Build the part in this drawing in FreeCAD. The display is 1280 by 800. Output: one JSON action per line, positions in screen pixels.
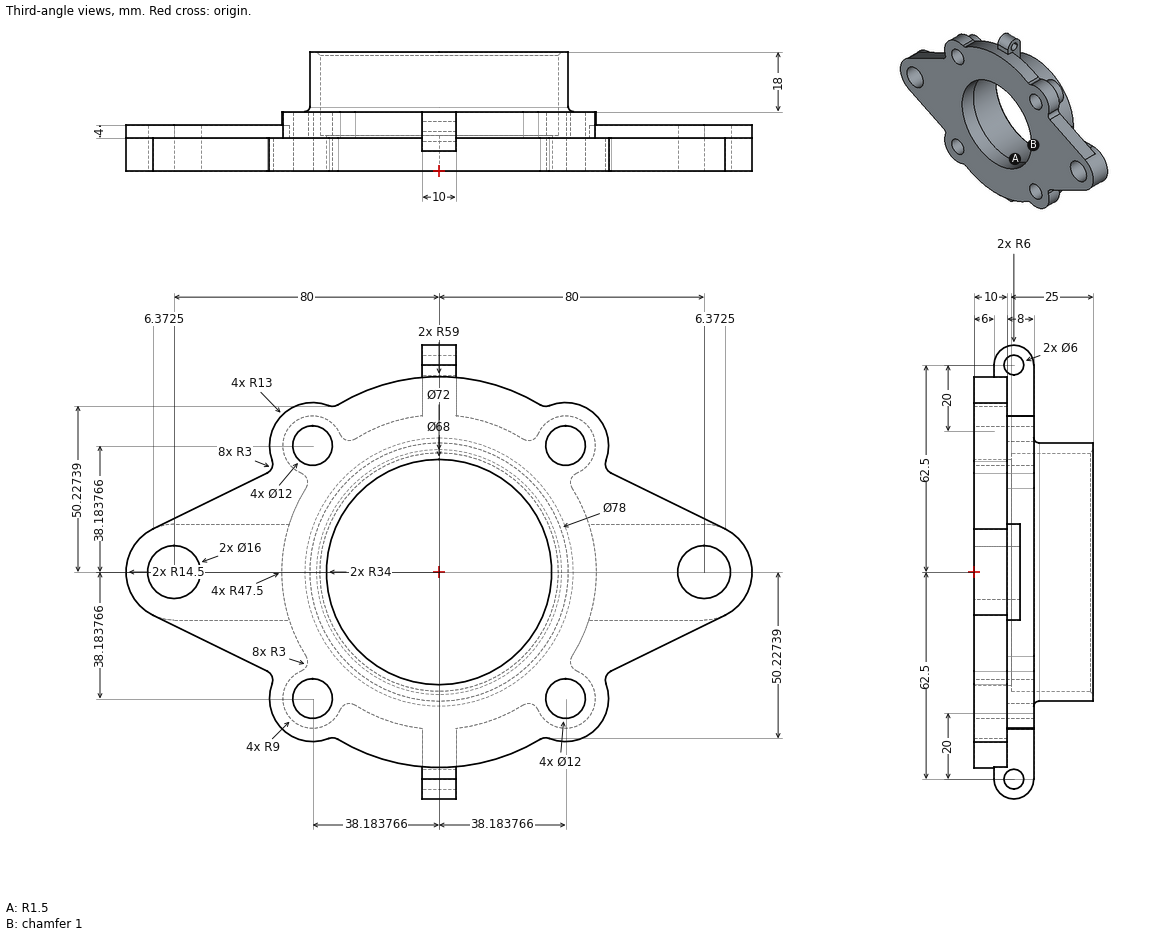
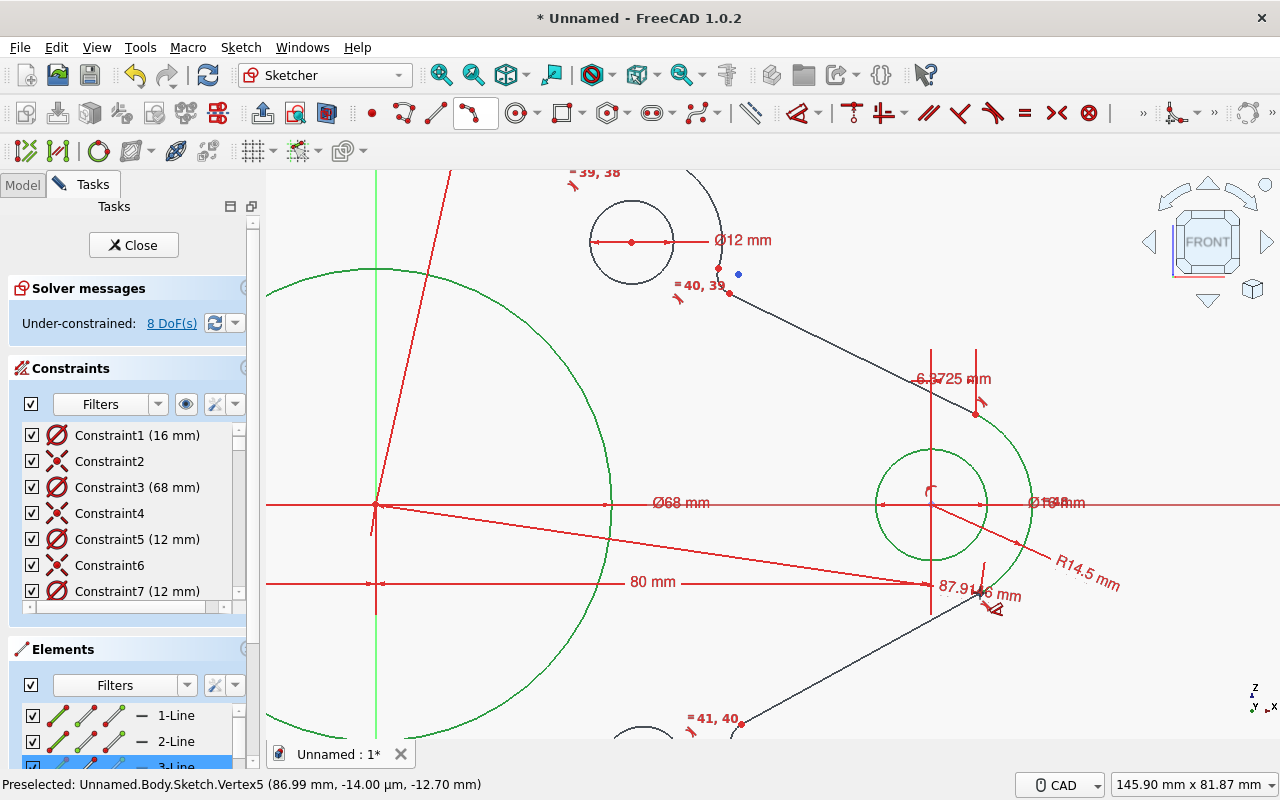
{"action": "left_click", "coordinate": [931, 505]}
{"action": "left_click", "coordinate": [956, 627]}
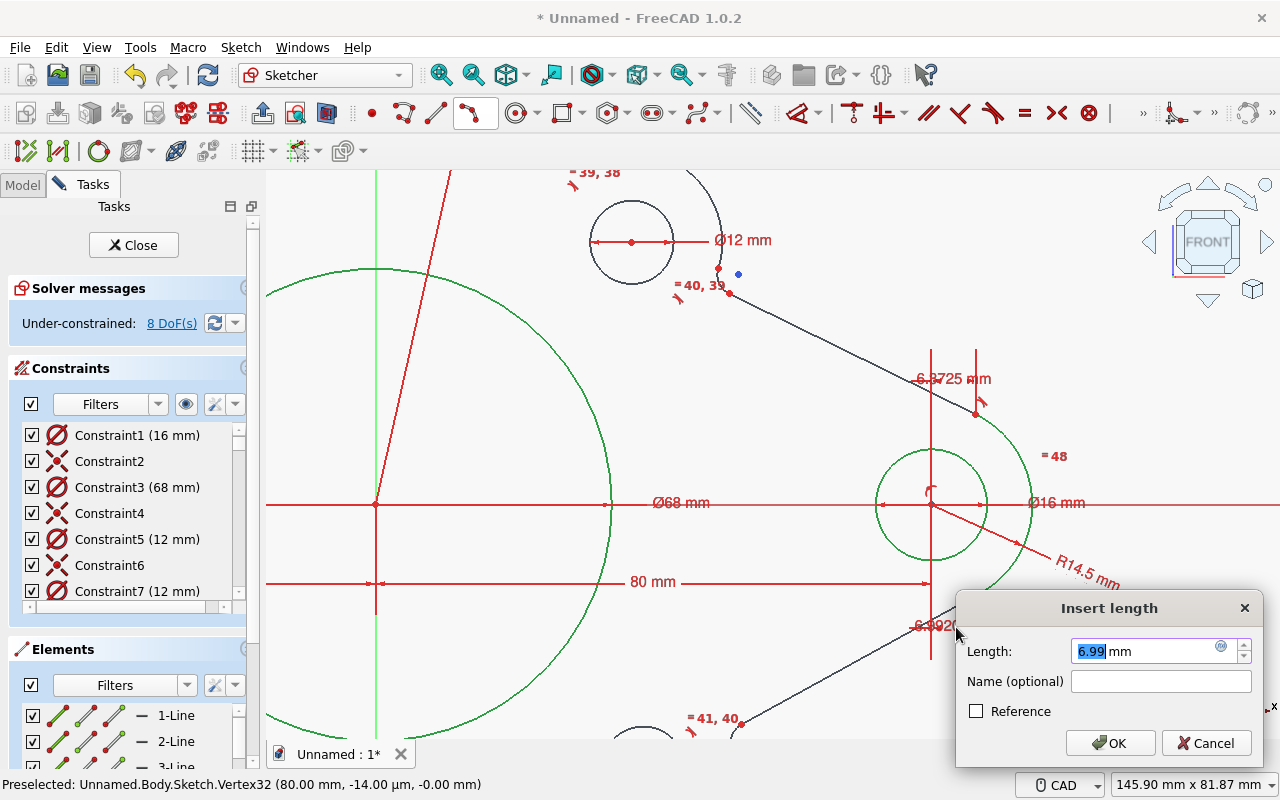
{"action": "type", "text": "6.3725"}
{"action": "key", "text": "Return"}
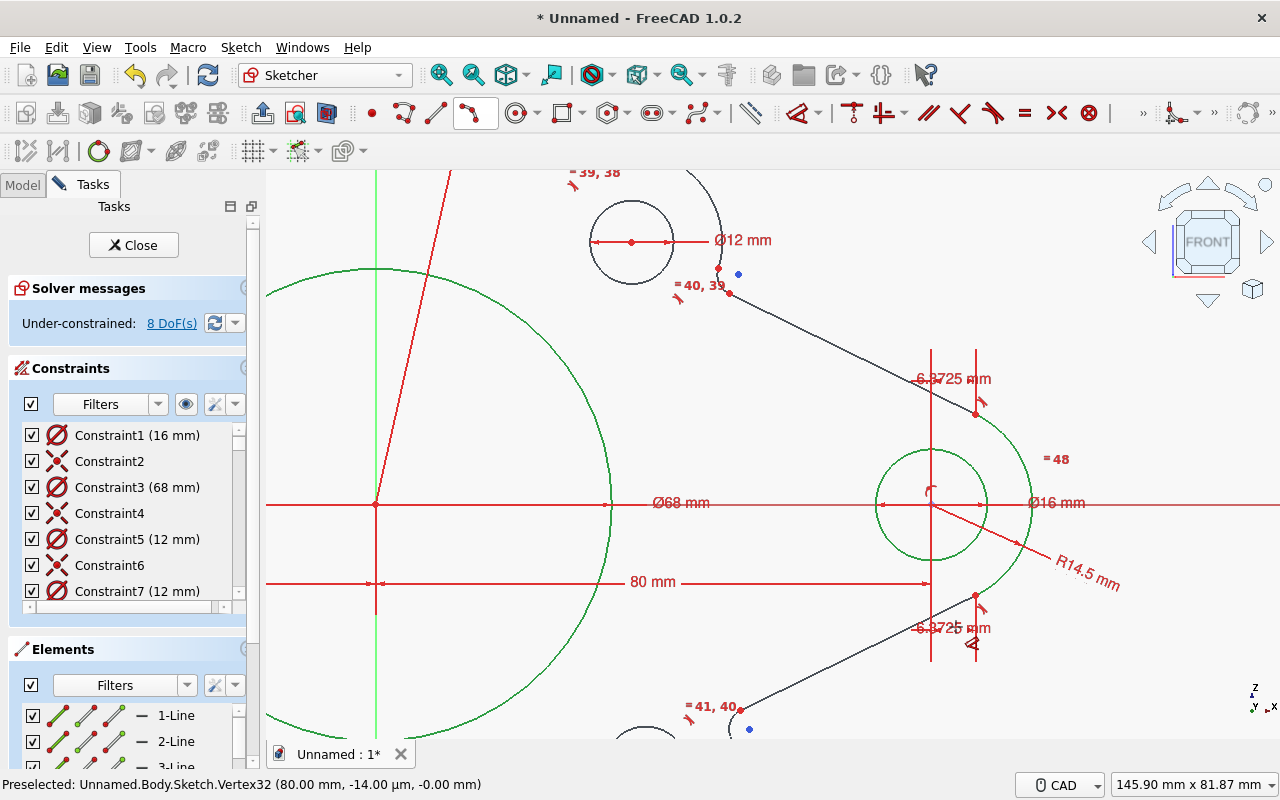
{"action": "scroll", "coordinate": [973, 413], "scroll_direction": "down", "scroll_amount": 4}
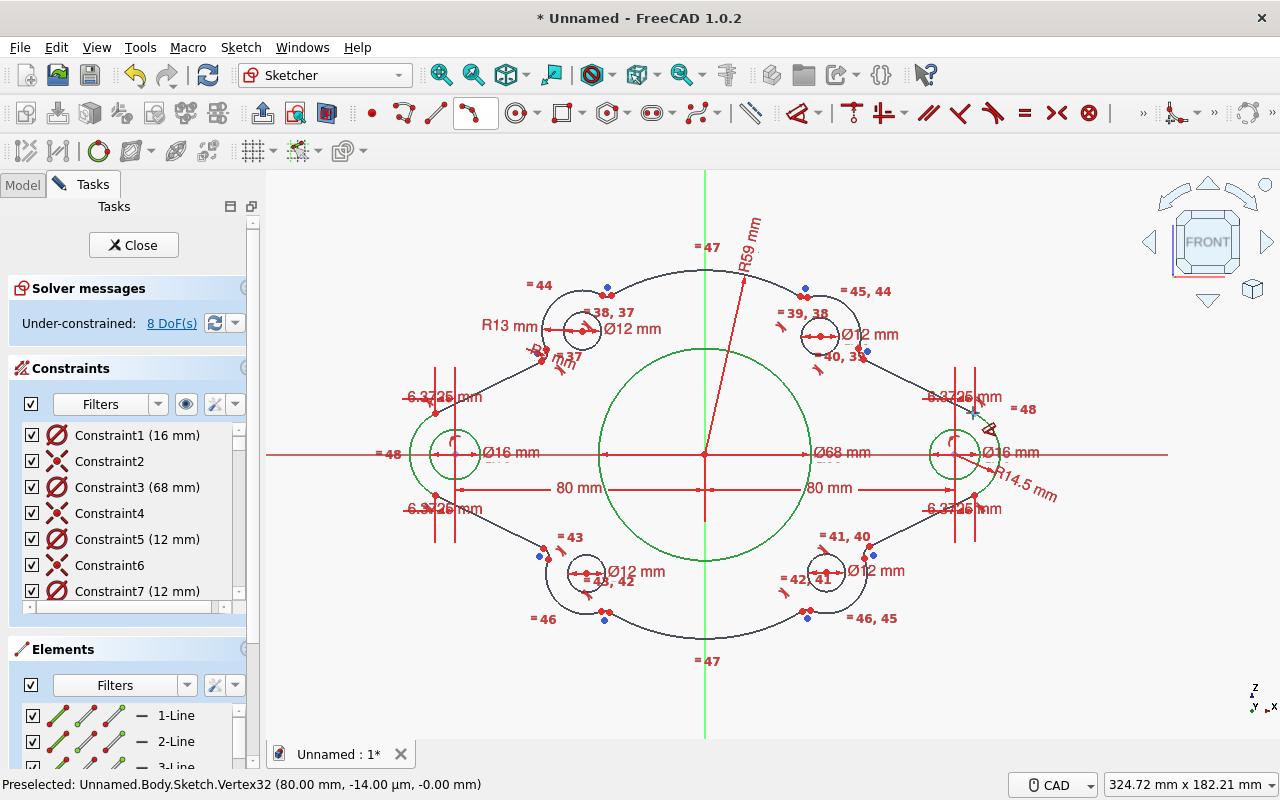
{"action": "scroll", "coordinate": [602, 296], "scroll_direction": "up", "scroll_amount": 2}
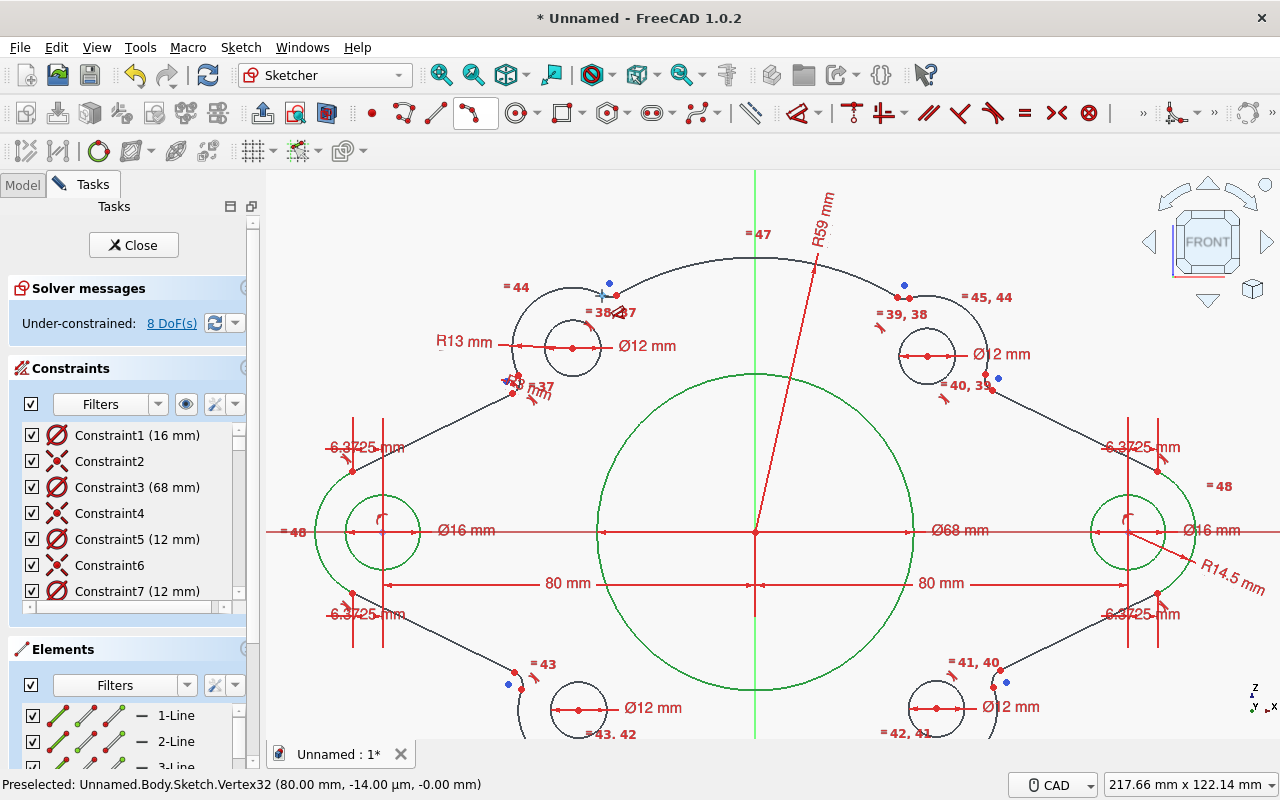
{"action": "left_click", "coordinate": [603, 295]}
{"action": "left_click", "coordinate": [569, 414]}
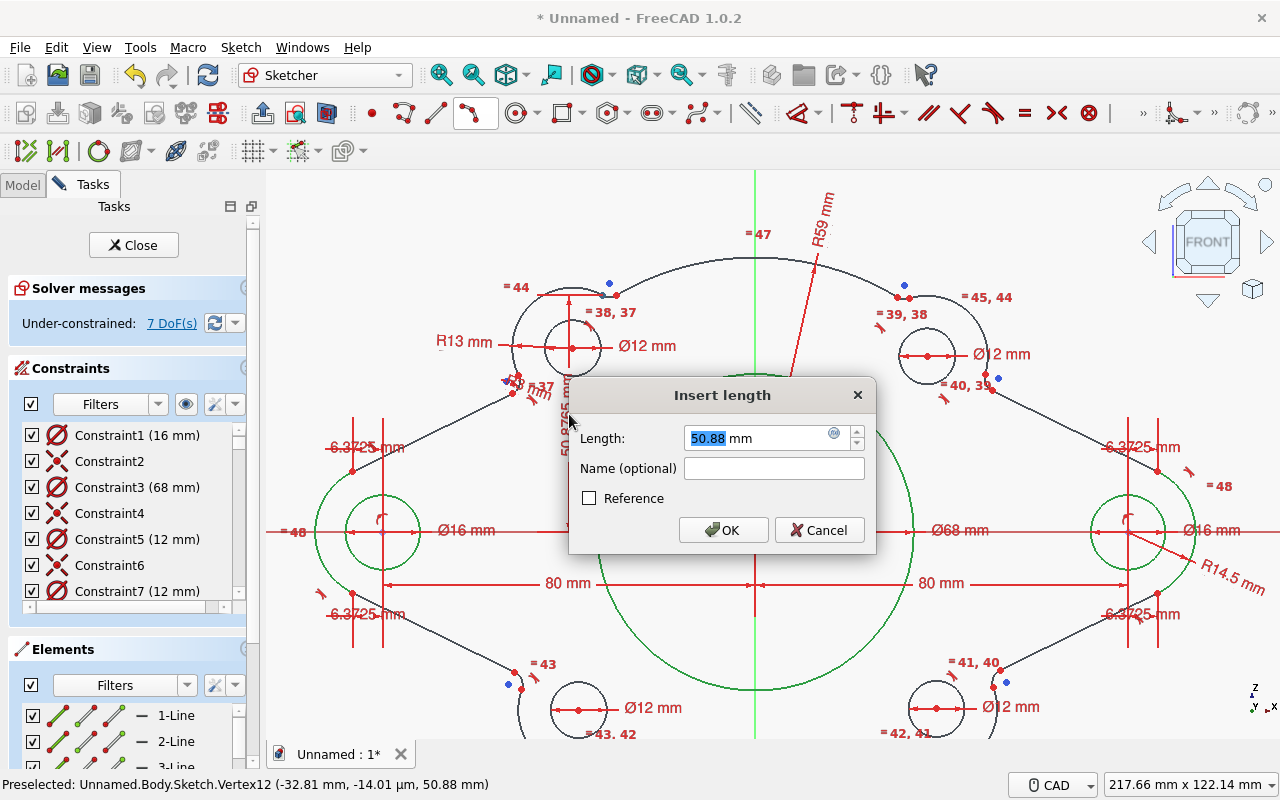
{"action": "type", "text": "50.22739"}
{"action": "key", "text": "Return"}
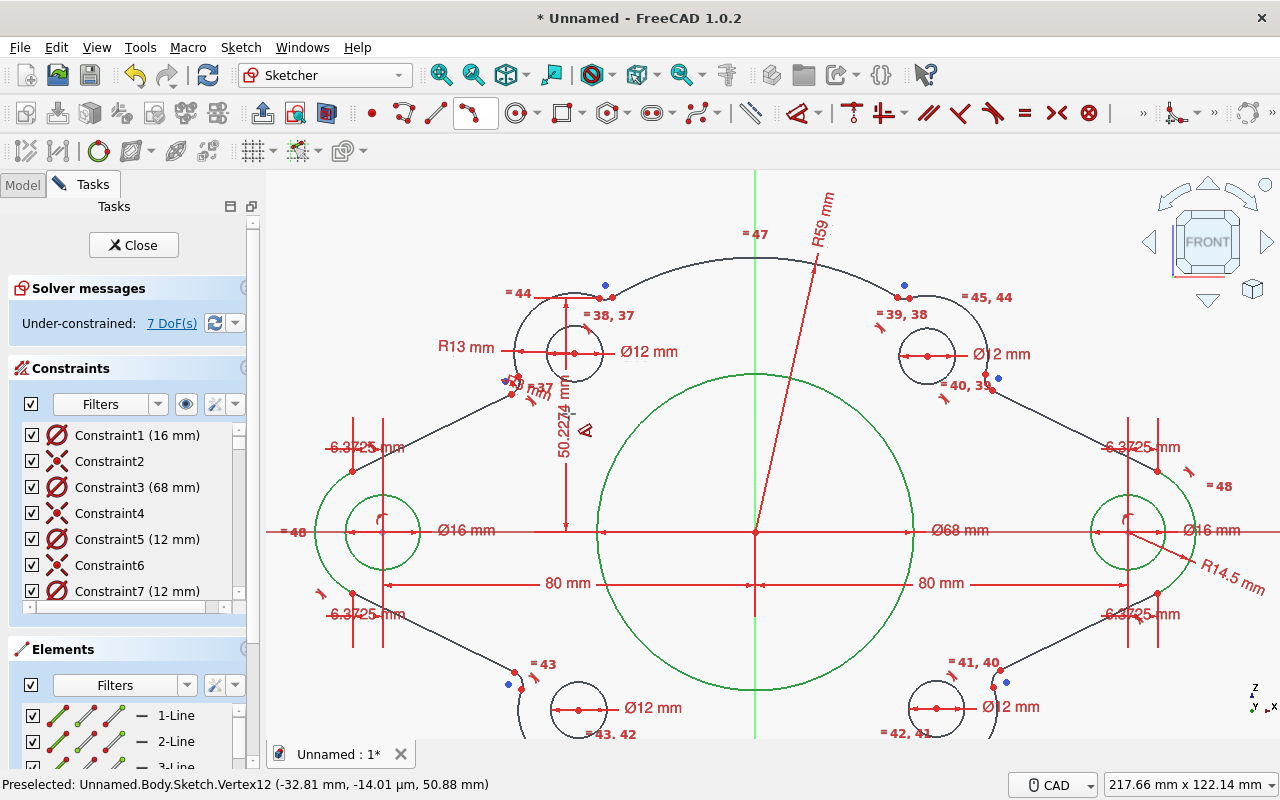
{"action": "left_click", "coordinate": [909, 299]}
{"action": "left_click", "coordinate": [943, 416]}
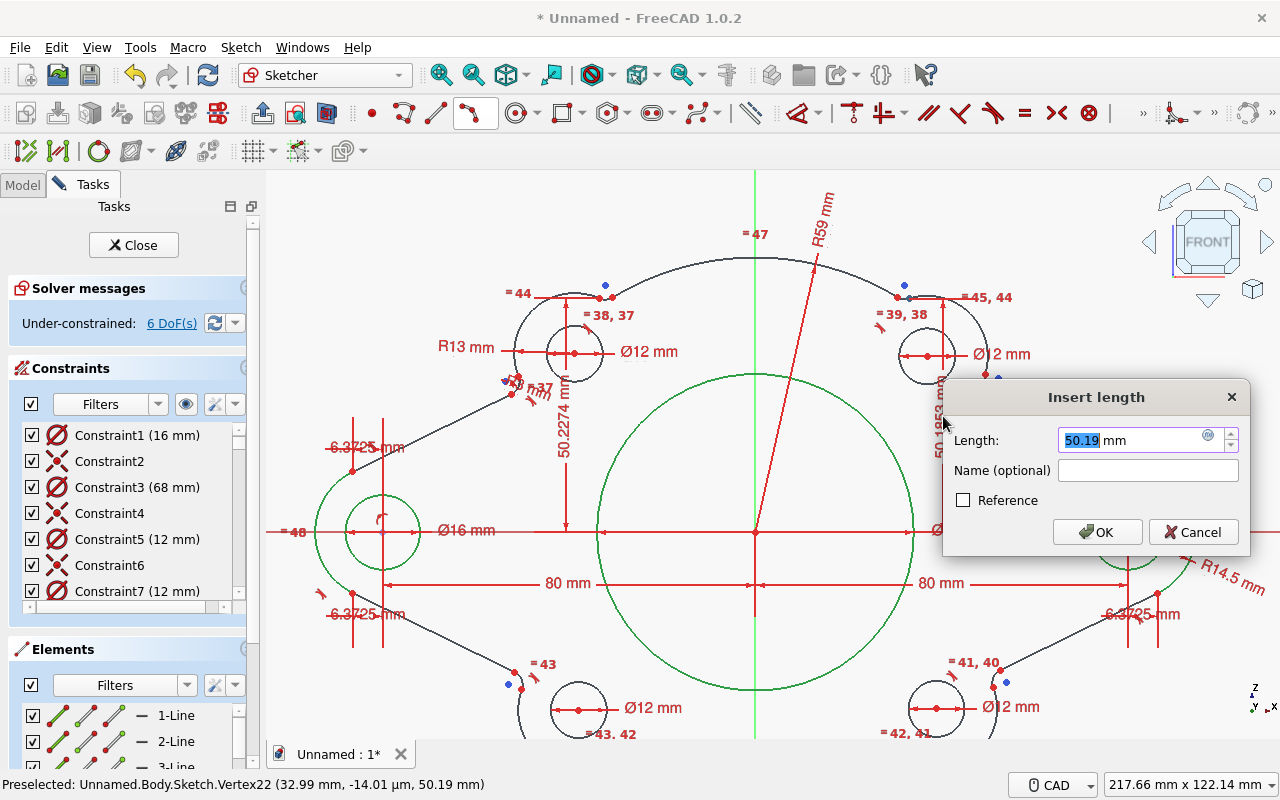
{"action": "type", "text": "50.22739"}
{"action": "key", "text": "Return"}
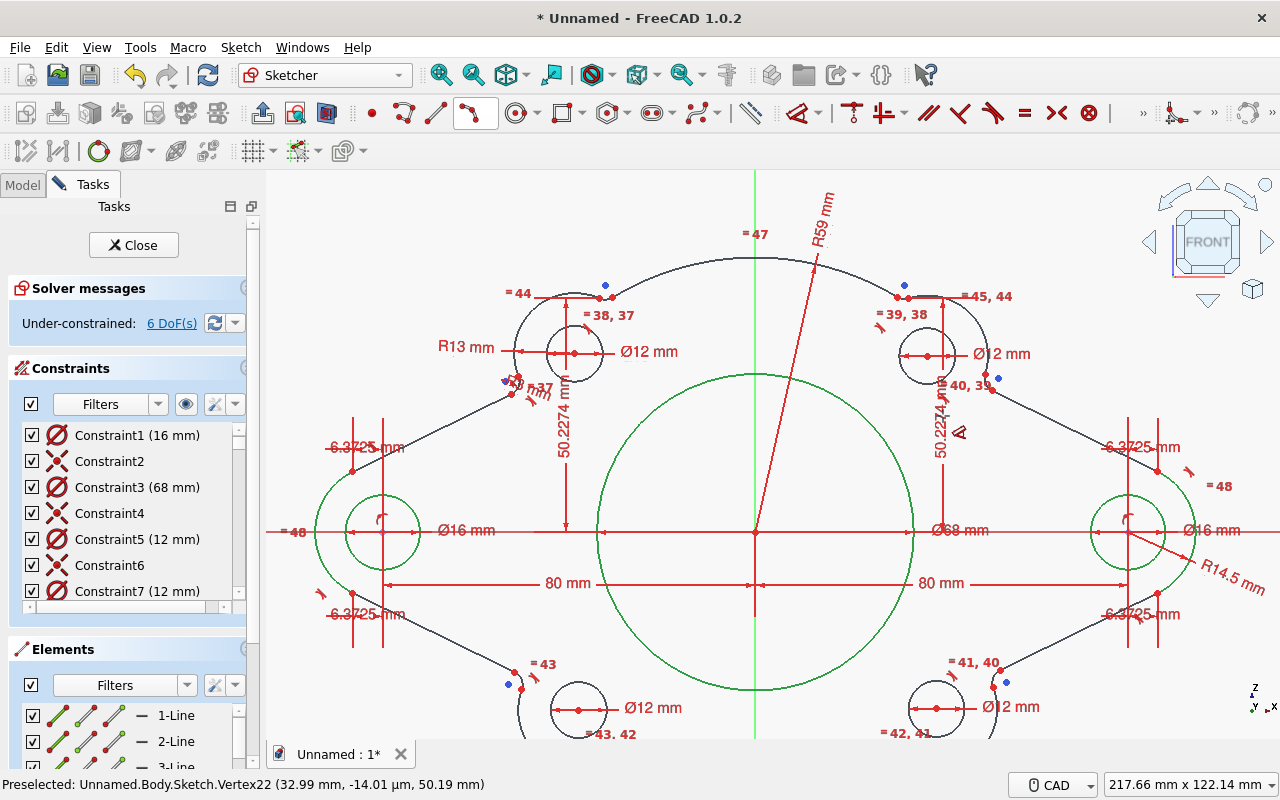
{"action": "scroll", "coordinate": [601, 296], "scroll_direction": "down", "scroll_amount": 2}